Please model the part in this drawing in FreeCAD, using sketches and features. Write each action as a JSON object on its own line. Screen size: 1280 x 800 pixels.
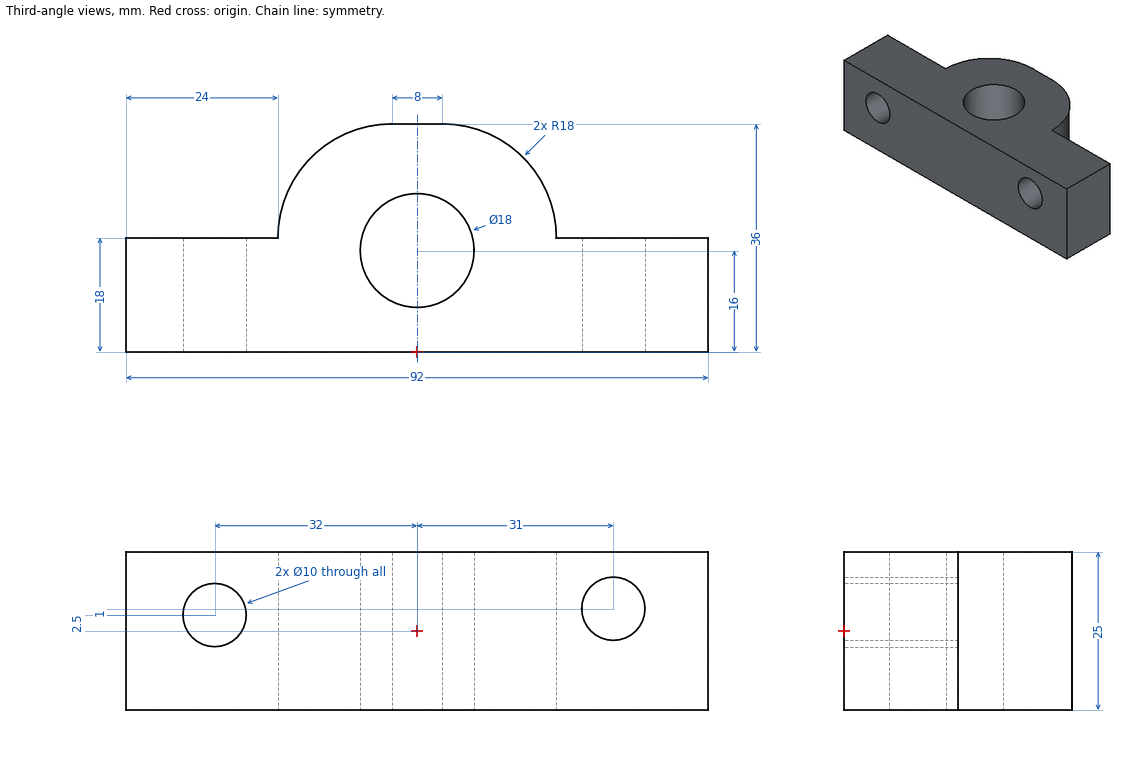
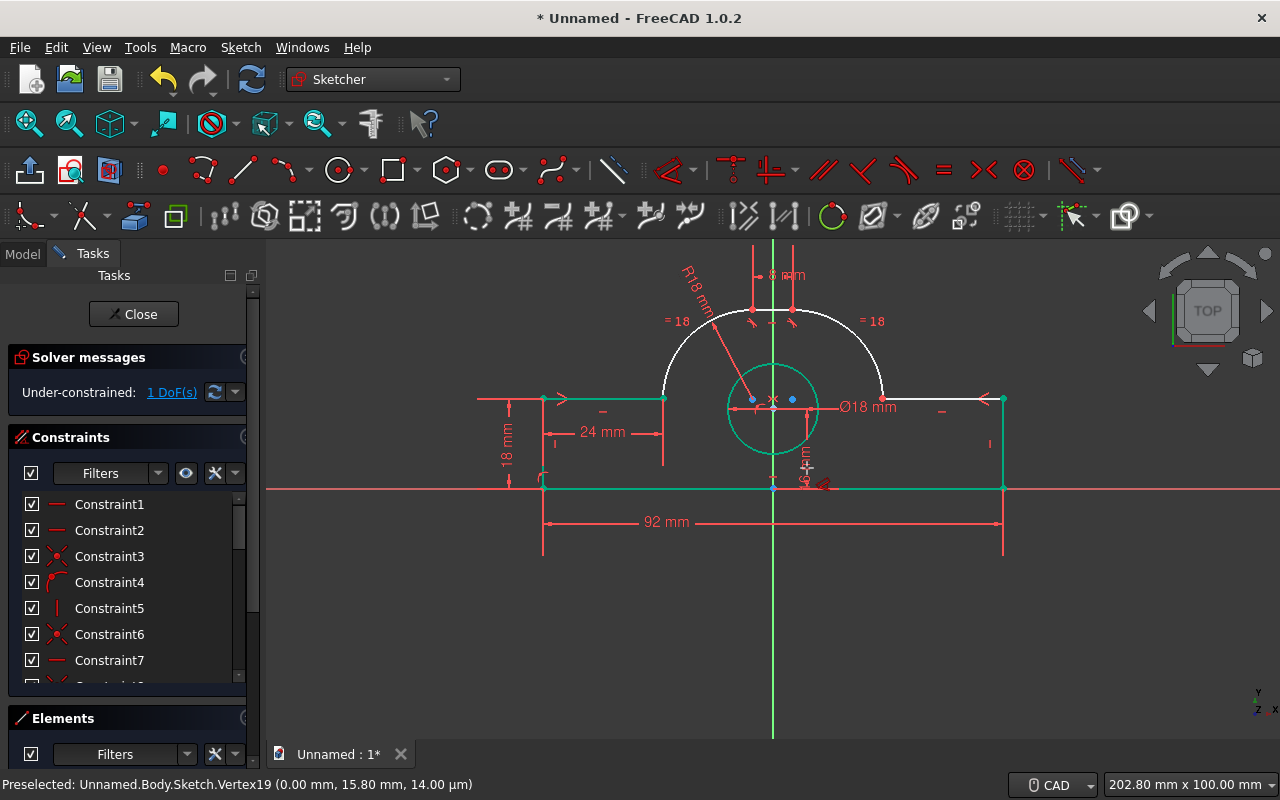
{"action": "left_click", "coordinate": [793, 310]}
{"action": "left_click", "coordinate": [827, 358]}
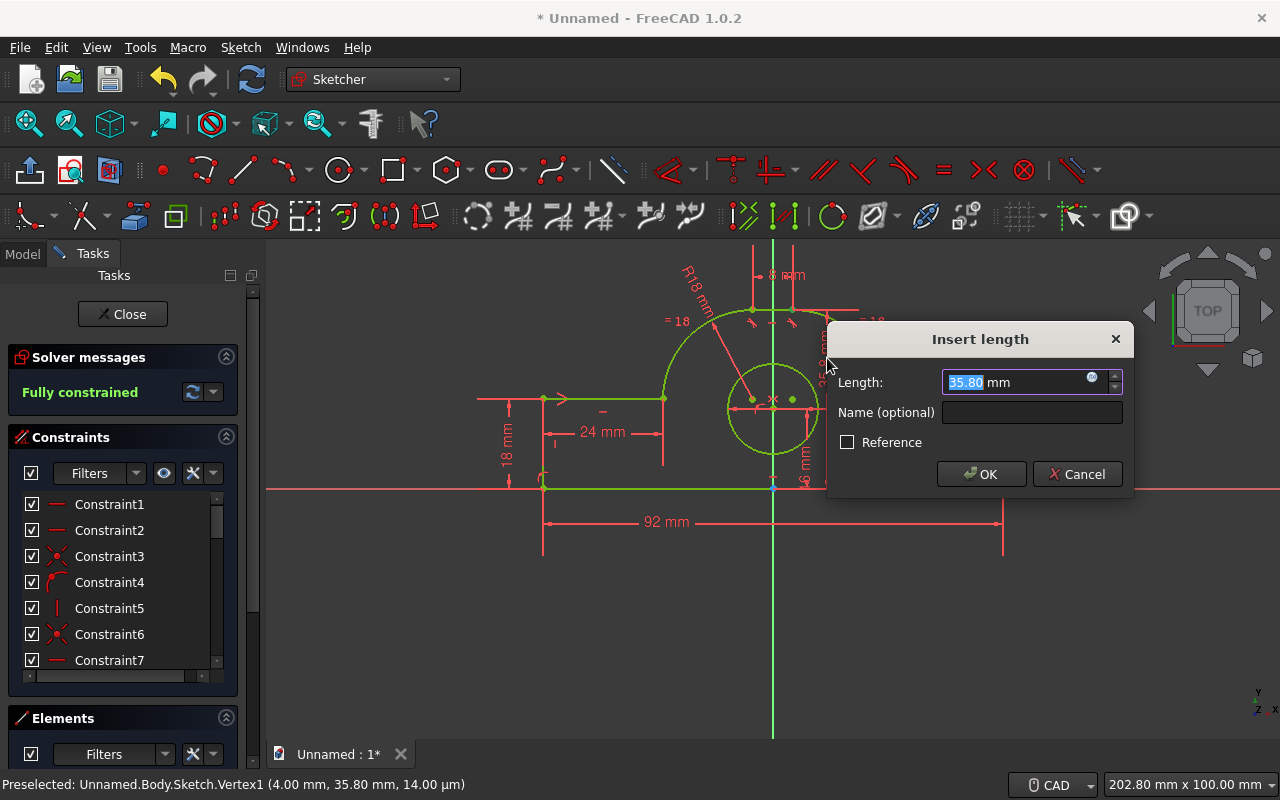
{"action": "type", "text": "36"}
{"action": "key", "text": "Return"}
{"action": "key", "text": "Escape"}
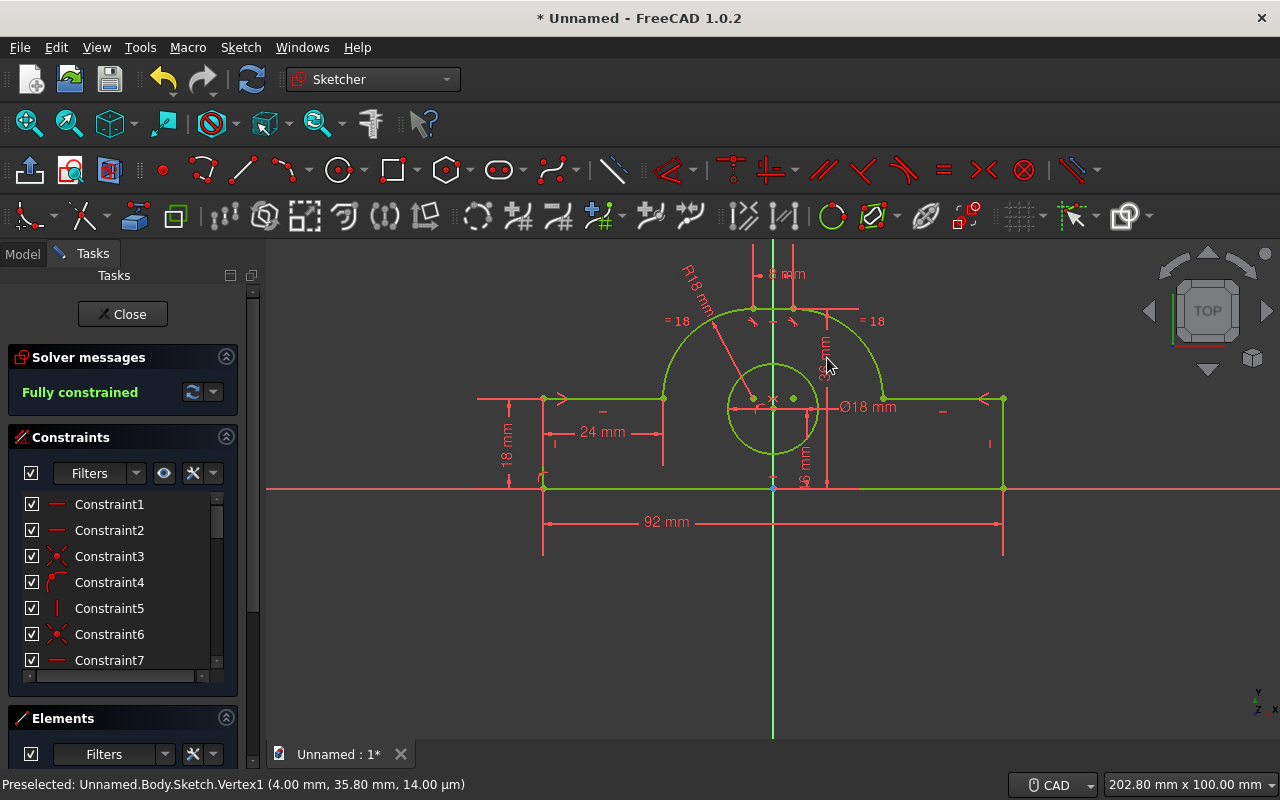
{"action": "left_click", "coordinate": [123, 314]}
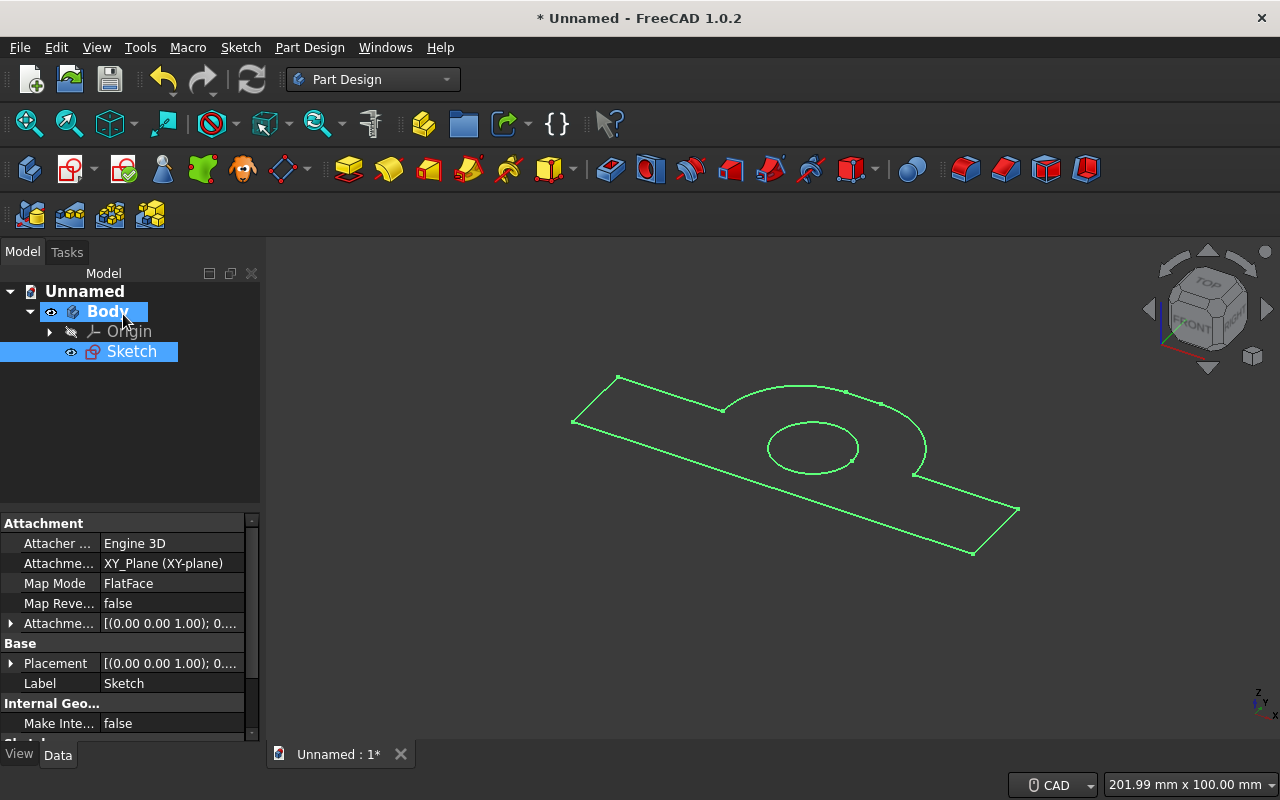
{"action": "left_click", "coordinate": [350, 170]}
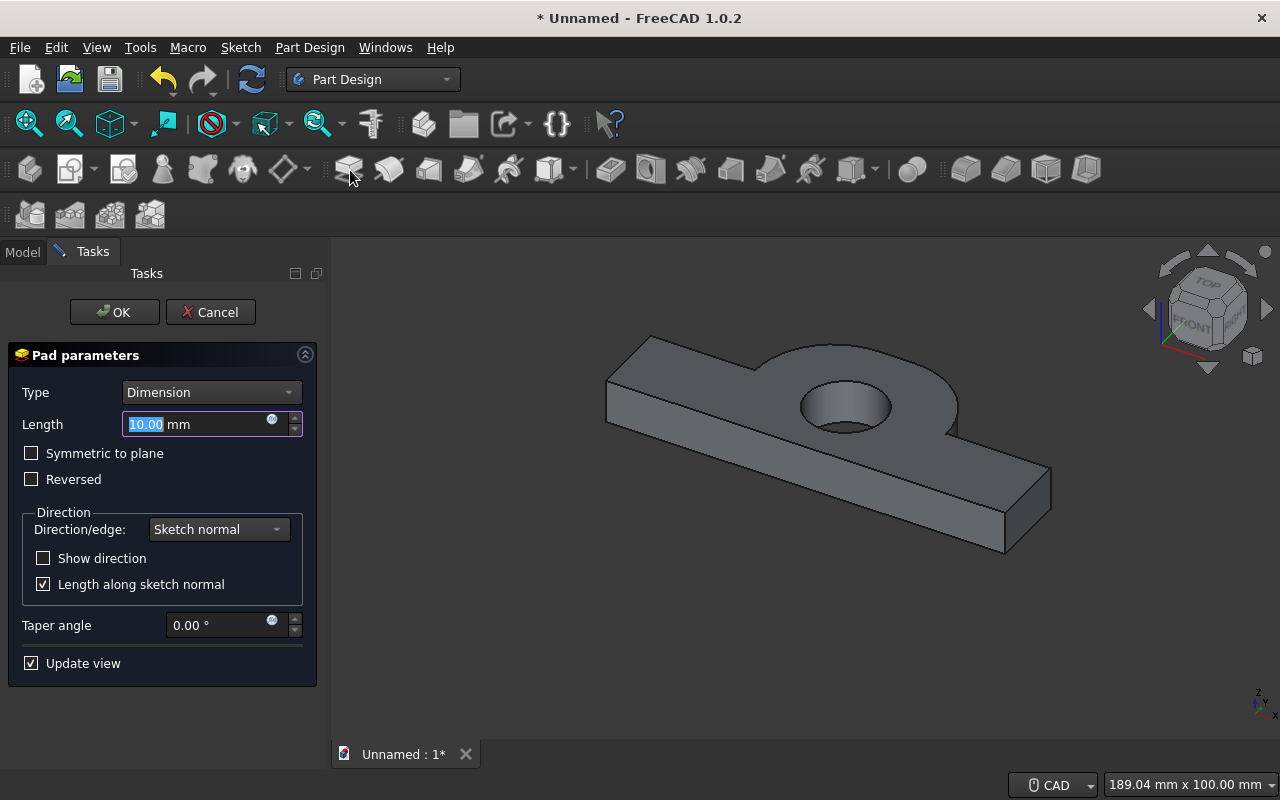
{"action": "type", "text": "25"}
{"action": "key", "text": "Tab"}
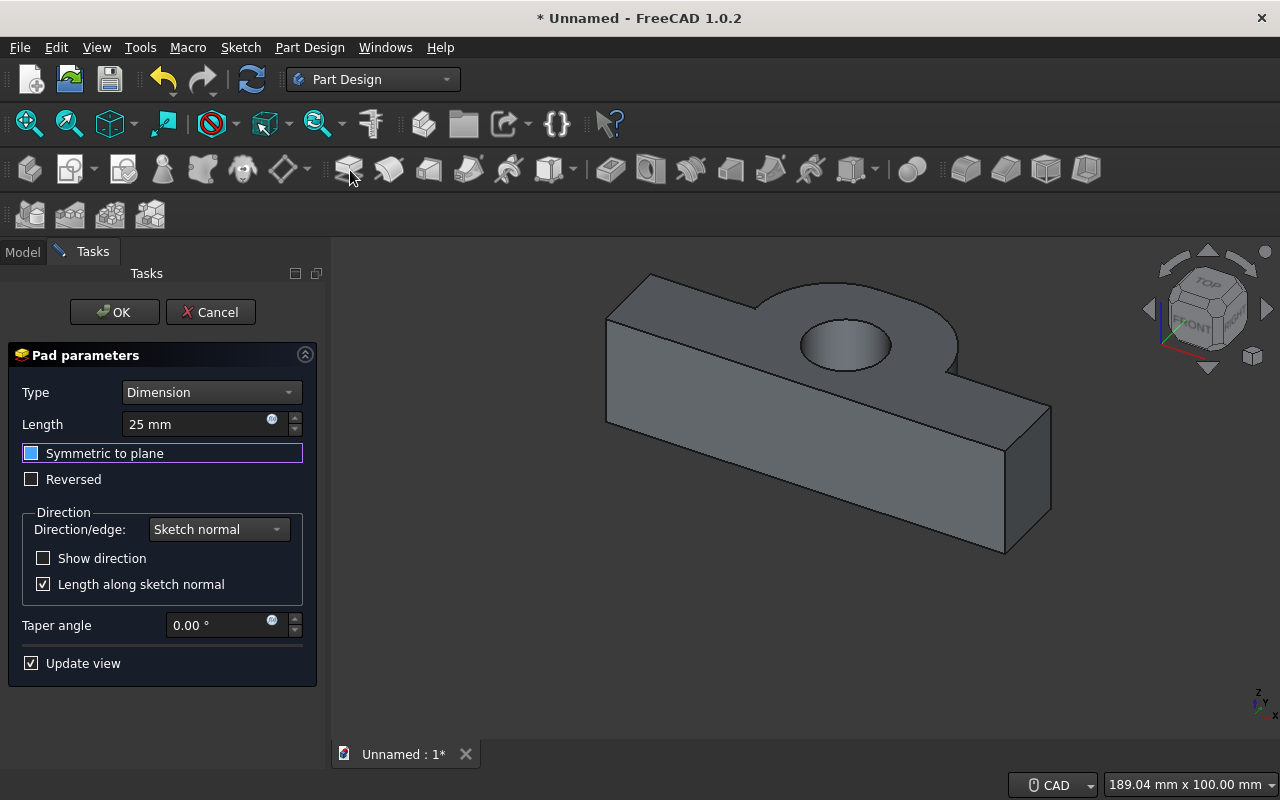
{"action": "left_click", "coordinate": [30, 453]}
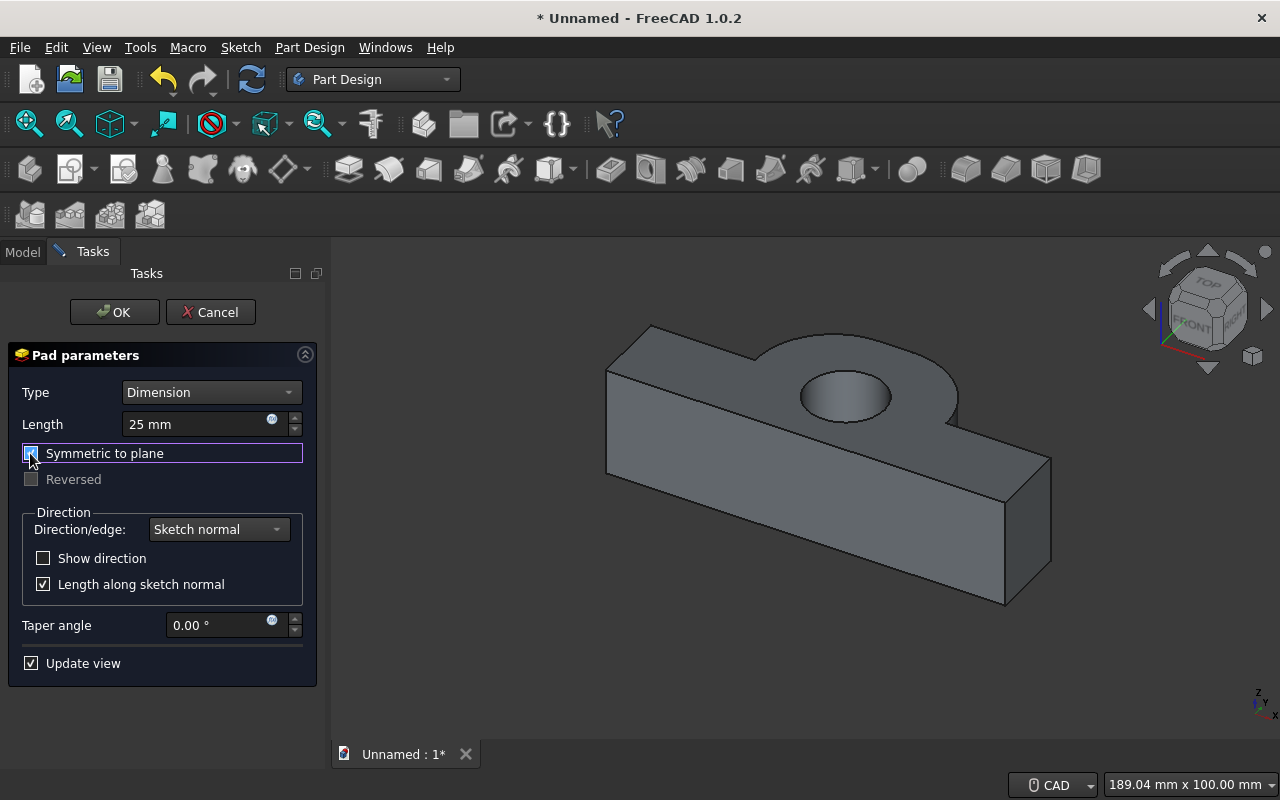
{"action": "left_click", "coordinate": [115, 312]}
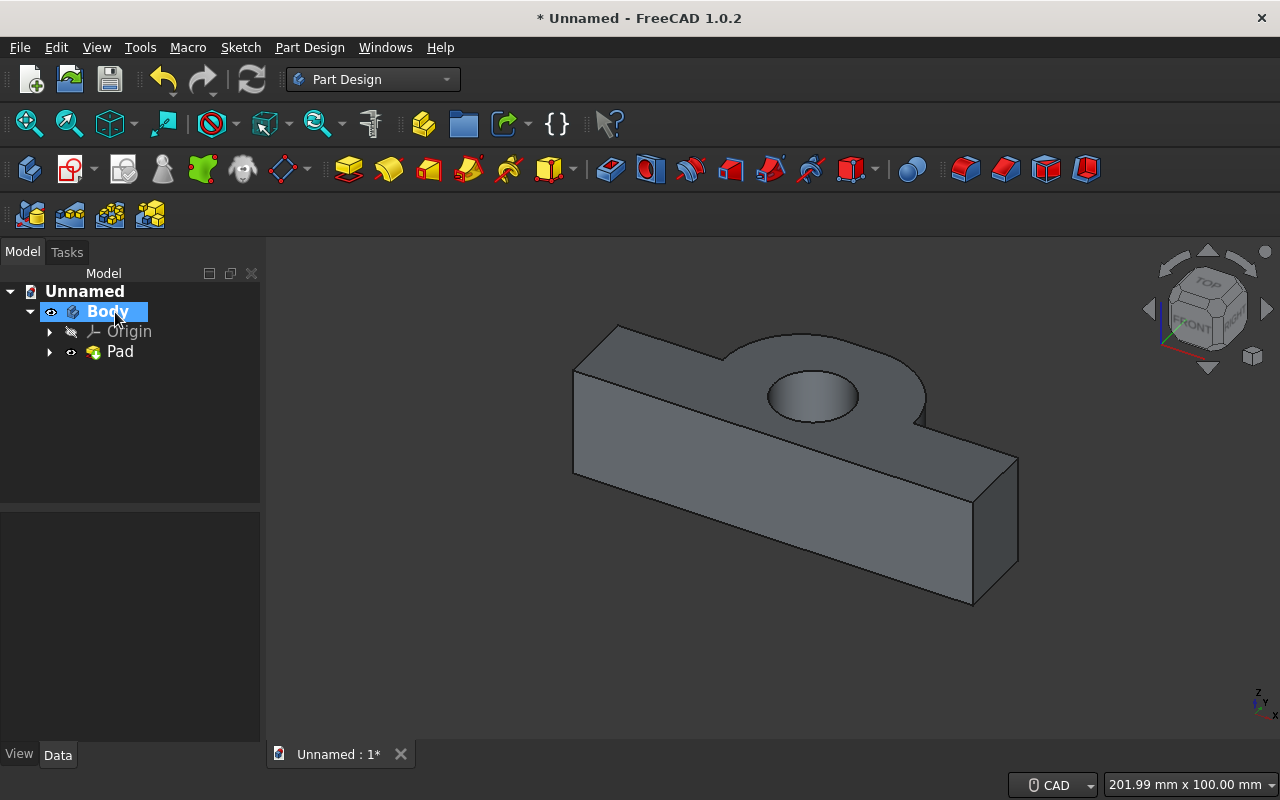
{"action": "key", "text": "4"}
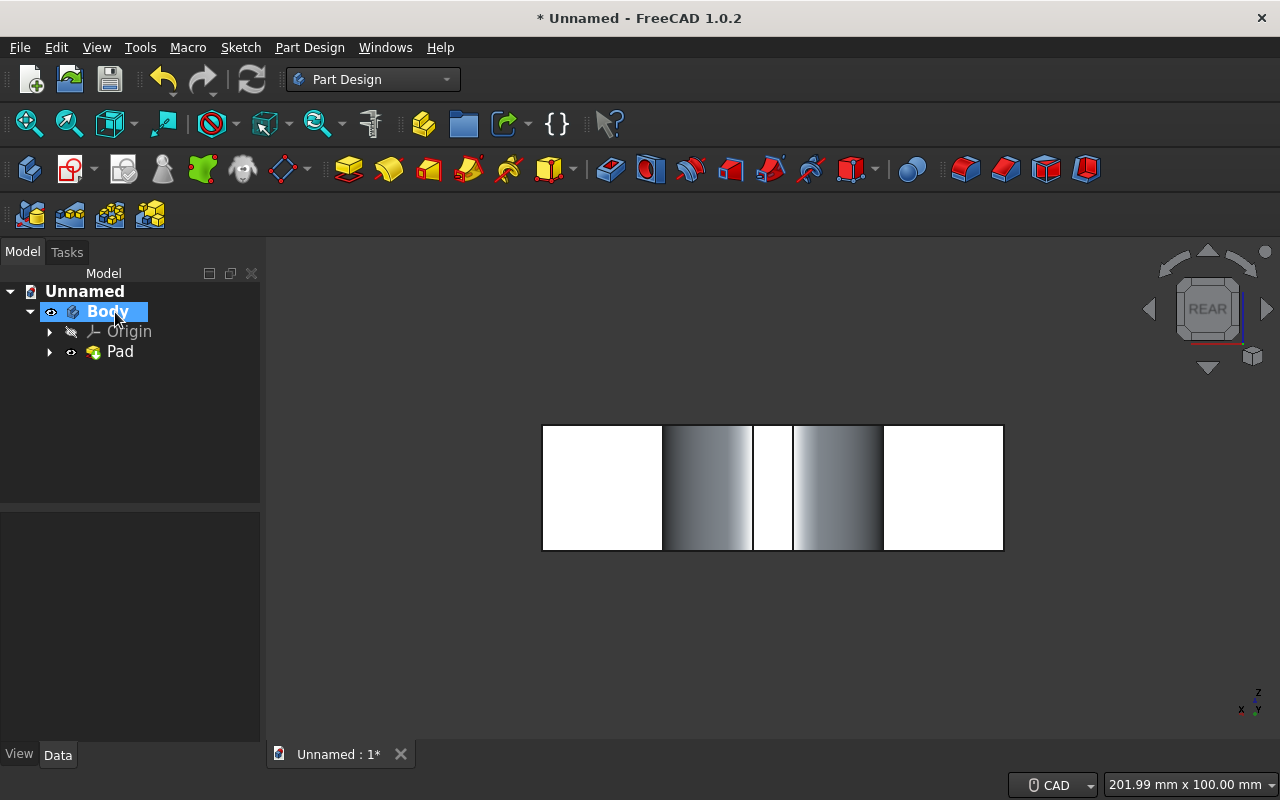
{"action": "left_click", "coordinate": [944, 487]}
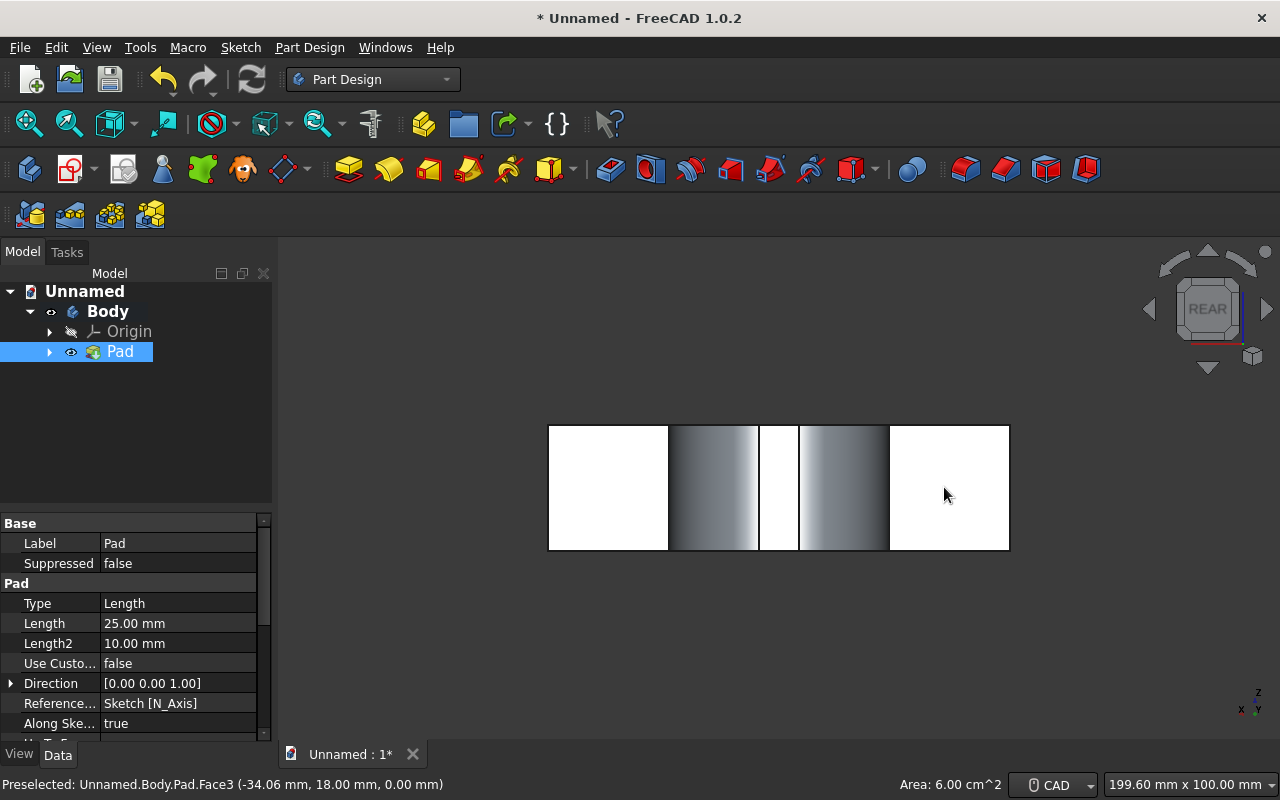
{"action": "left_click", "coordinate": [70, 170]}